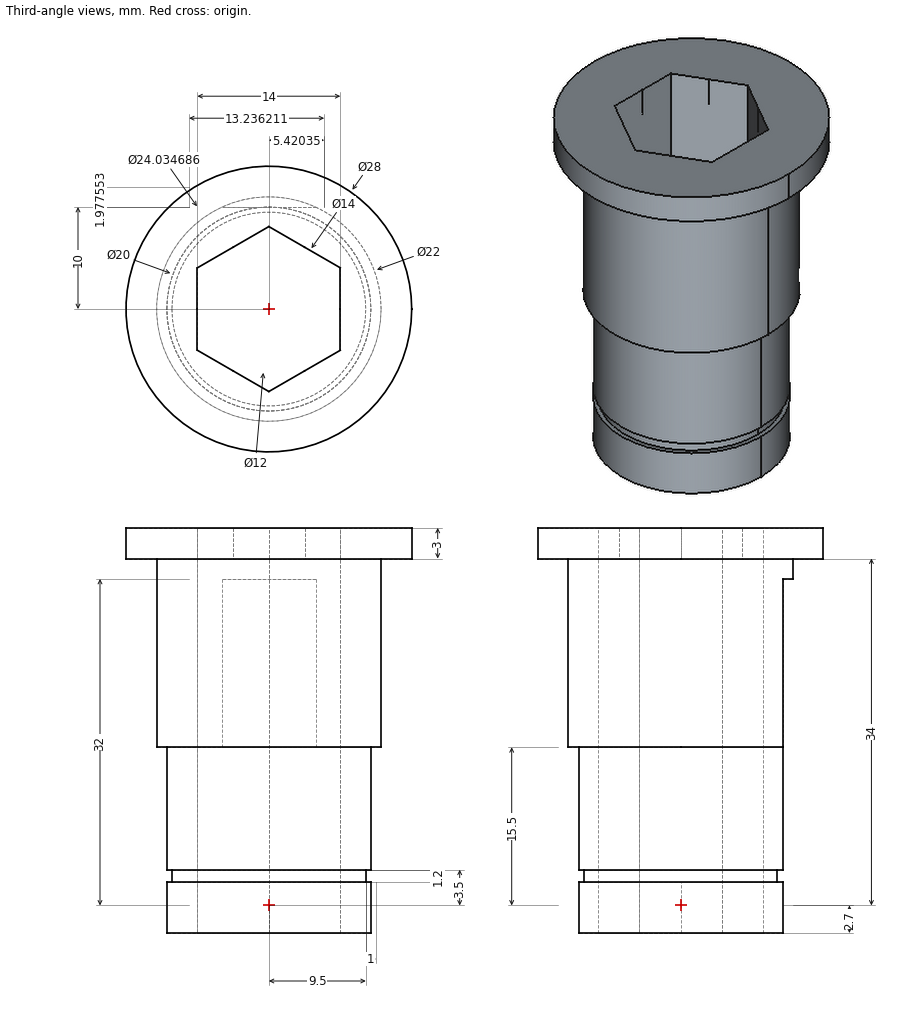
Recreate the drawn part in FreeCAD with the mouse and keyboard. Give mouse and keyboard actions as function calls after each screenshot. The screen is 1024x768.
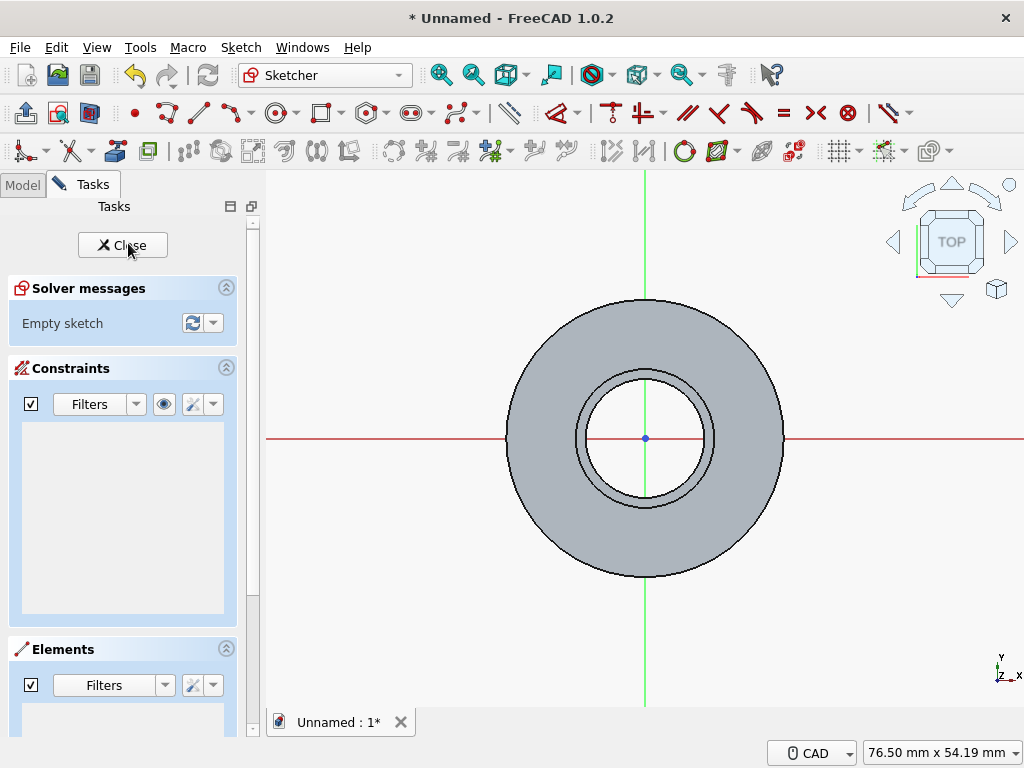
click(90, 114)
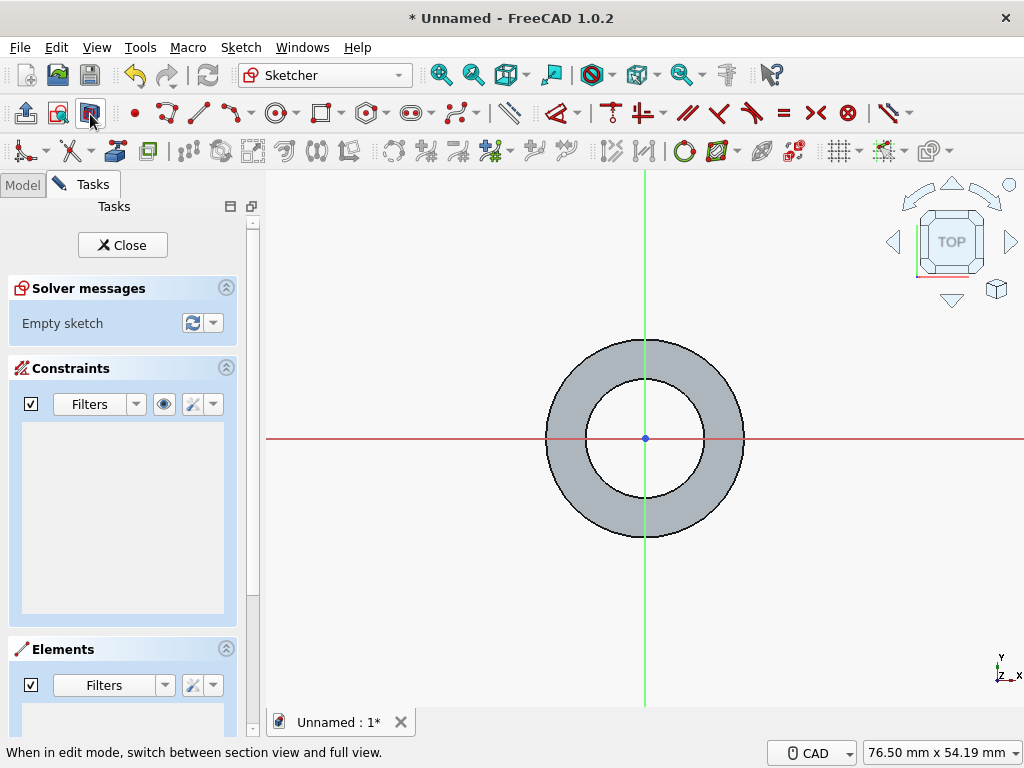
scroll(666, 345, up, 5)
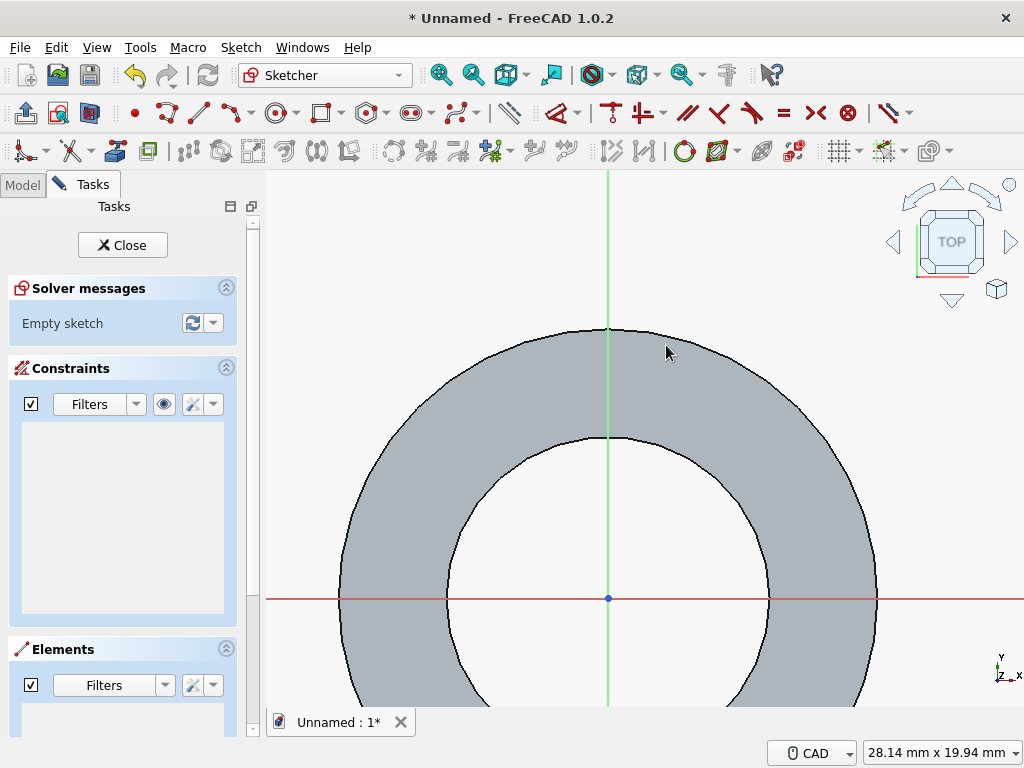
click(322, 114)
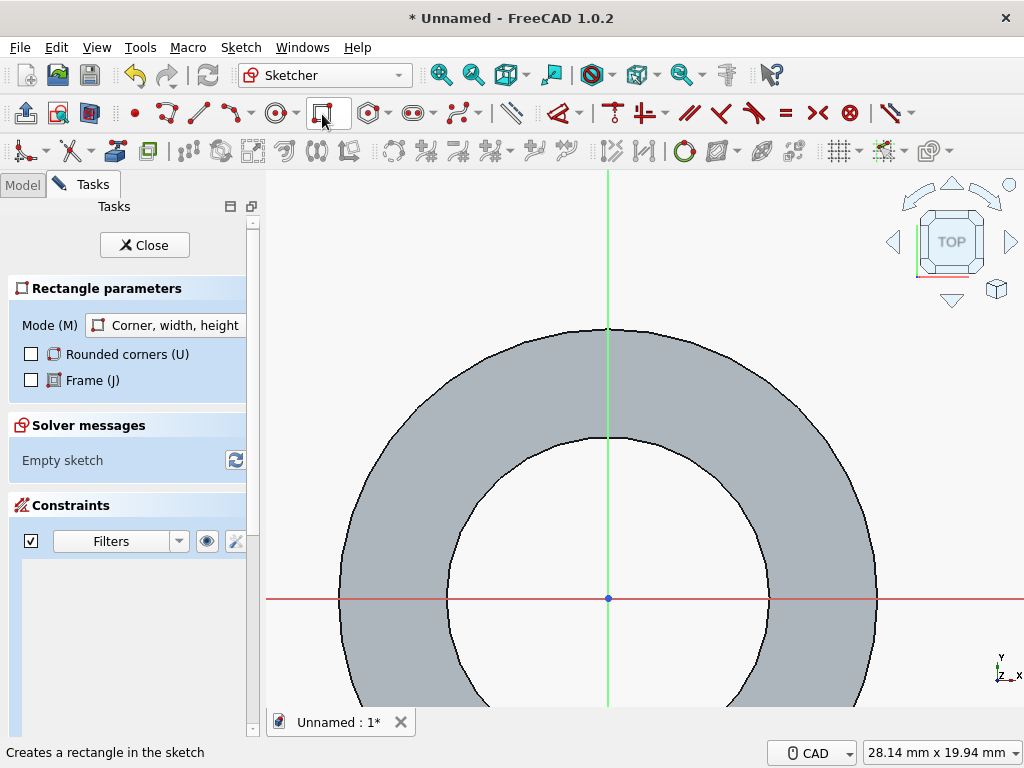
click(397, 276)
click(754, 329)
key(Escape)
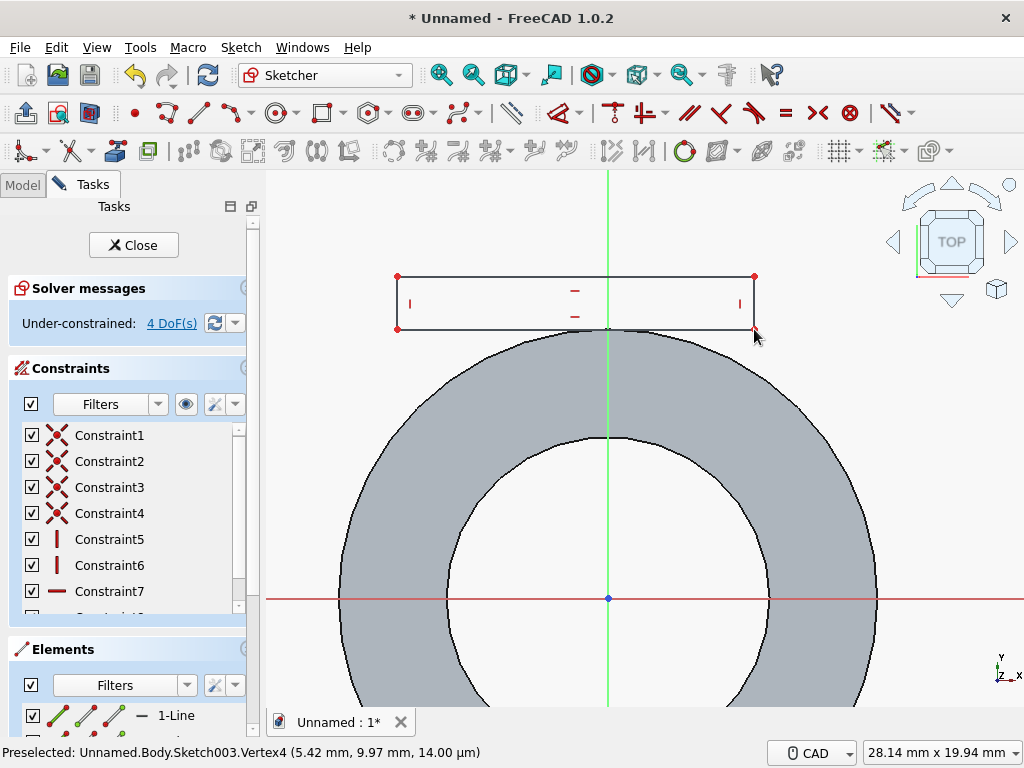
click(558, 114)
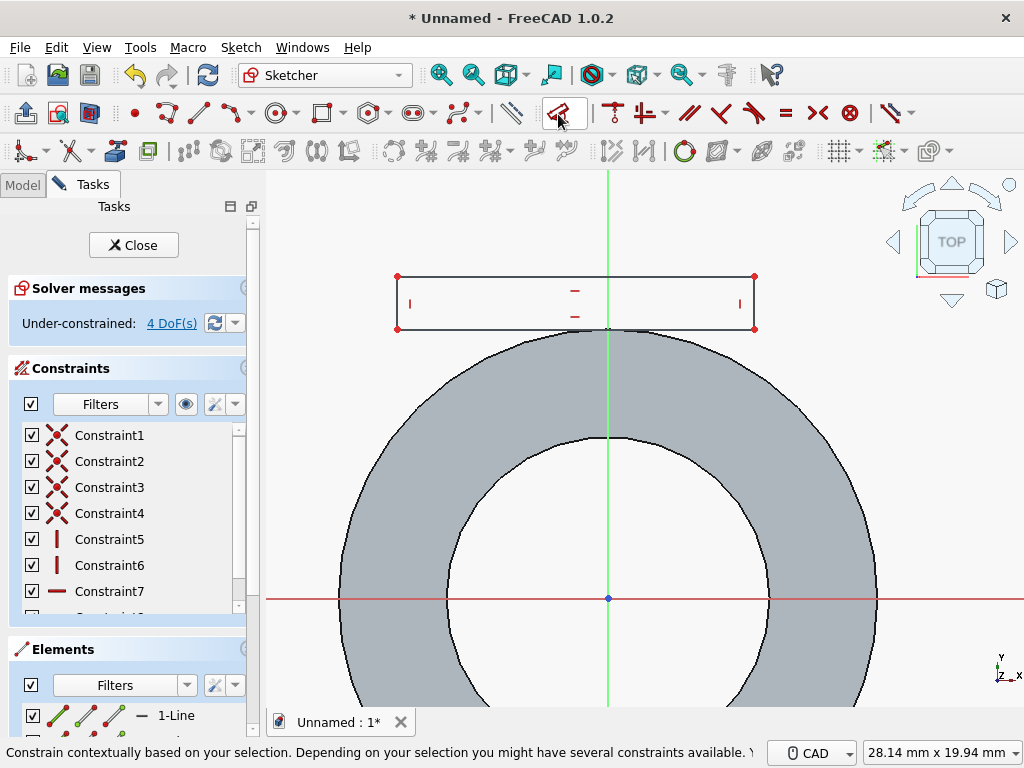
click(397, 330)
click(363, 464)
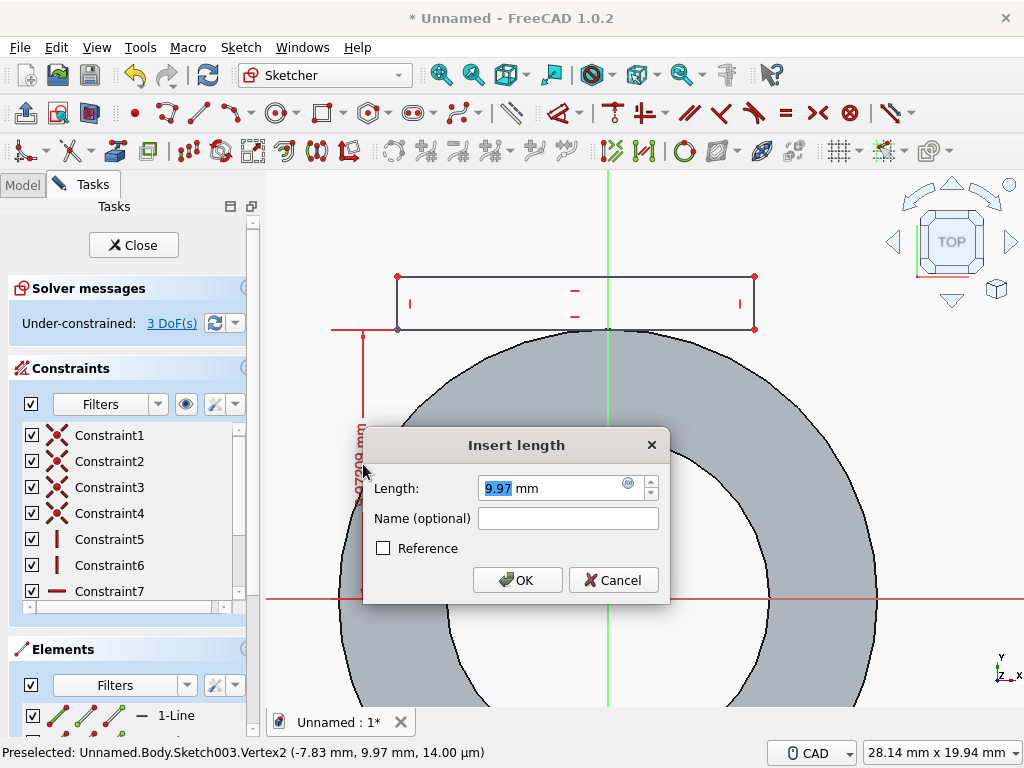
text(10)
key(Return)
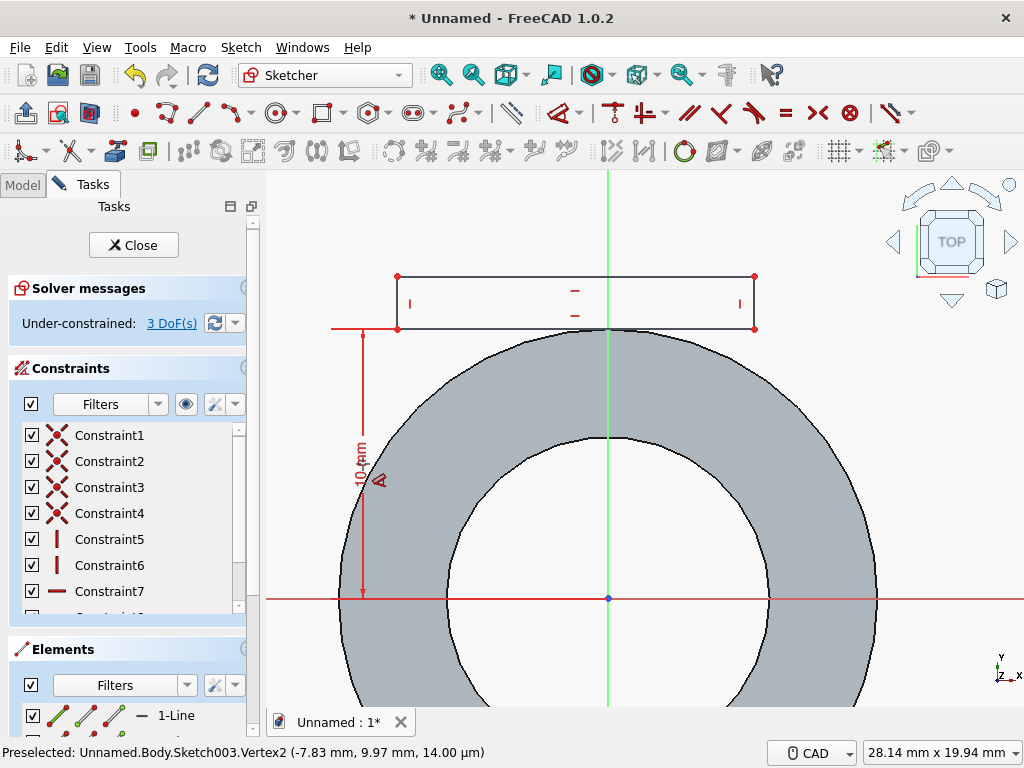
click(397, 293)
click(363, 303)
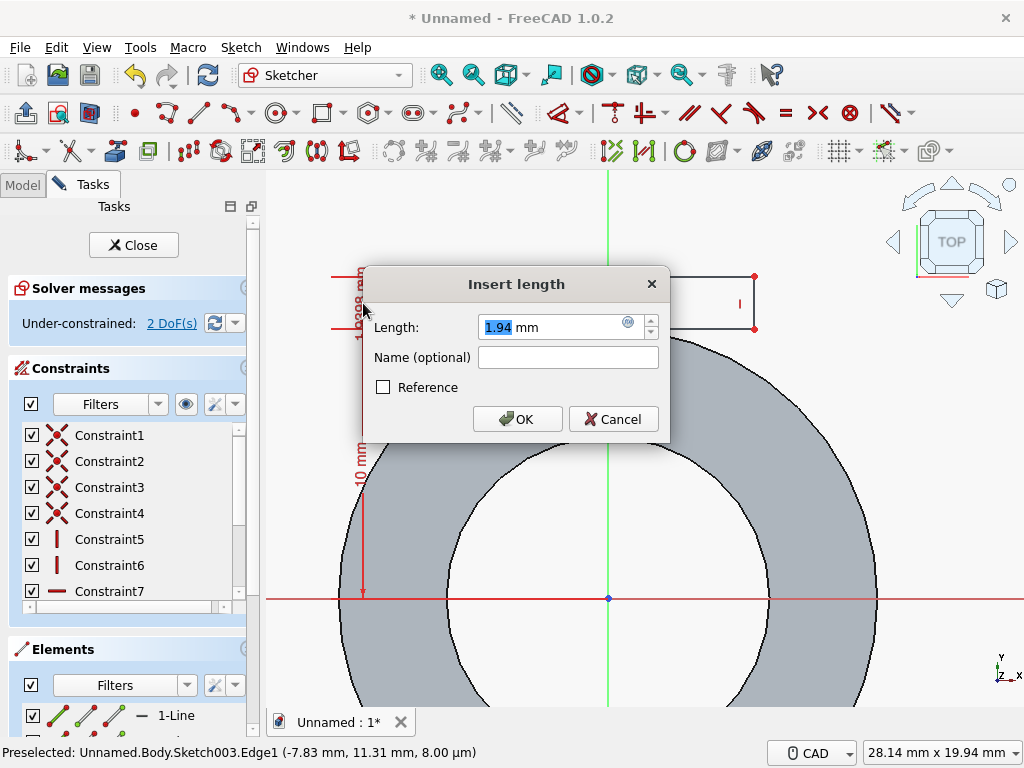
text(1.977553)
key(Return)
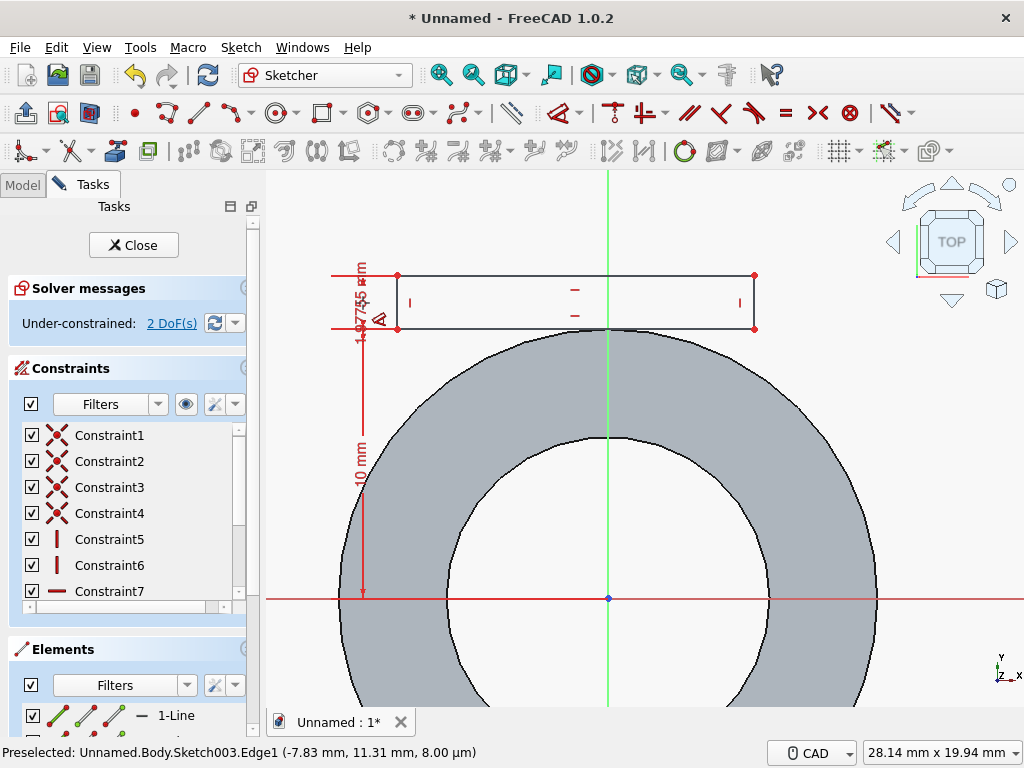
click(754, 329)
click(681, 633)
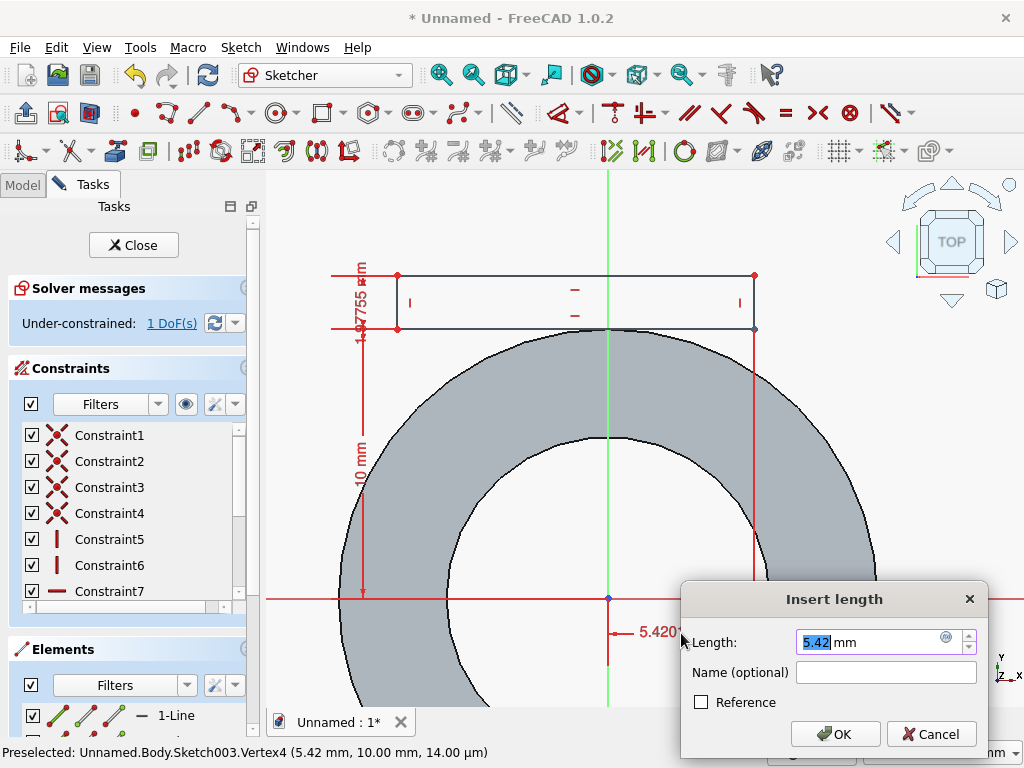
text(5.42035)
key(Return)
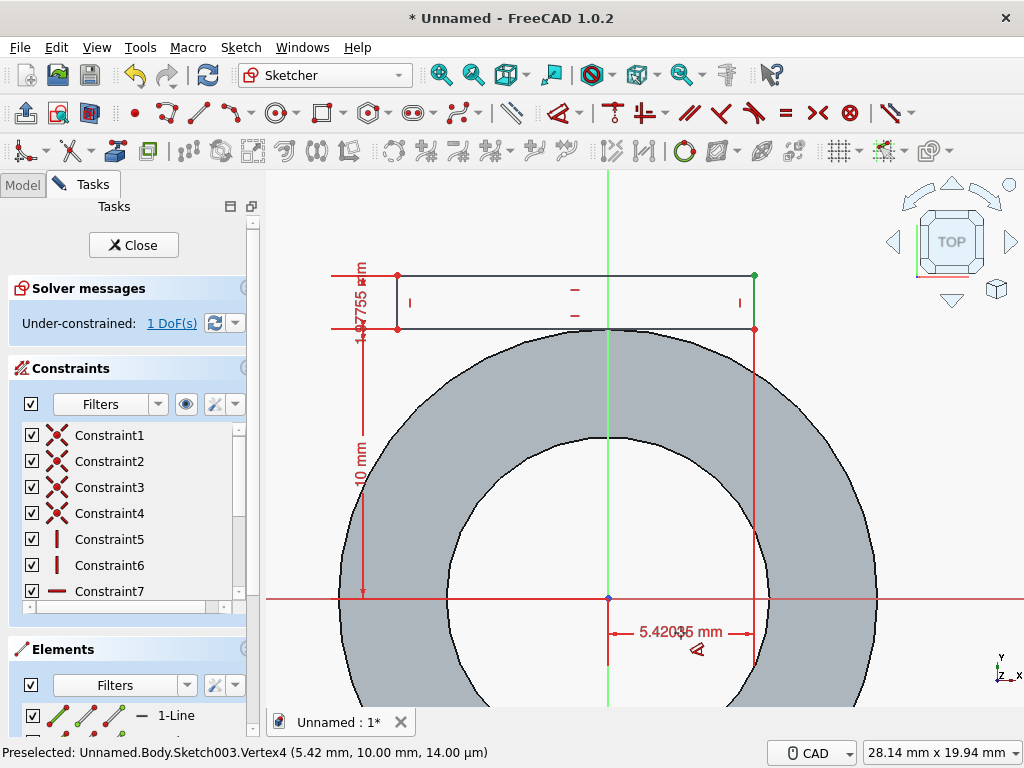
click(504, 329)
click(576, 295)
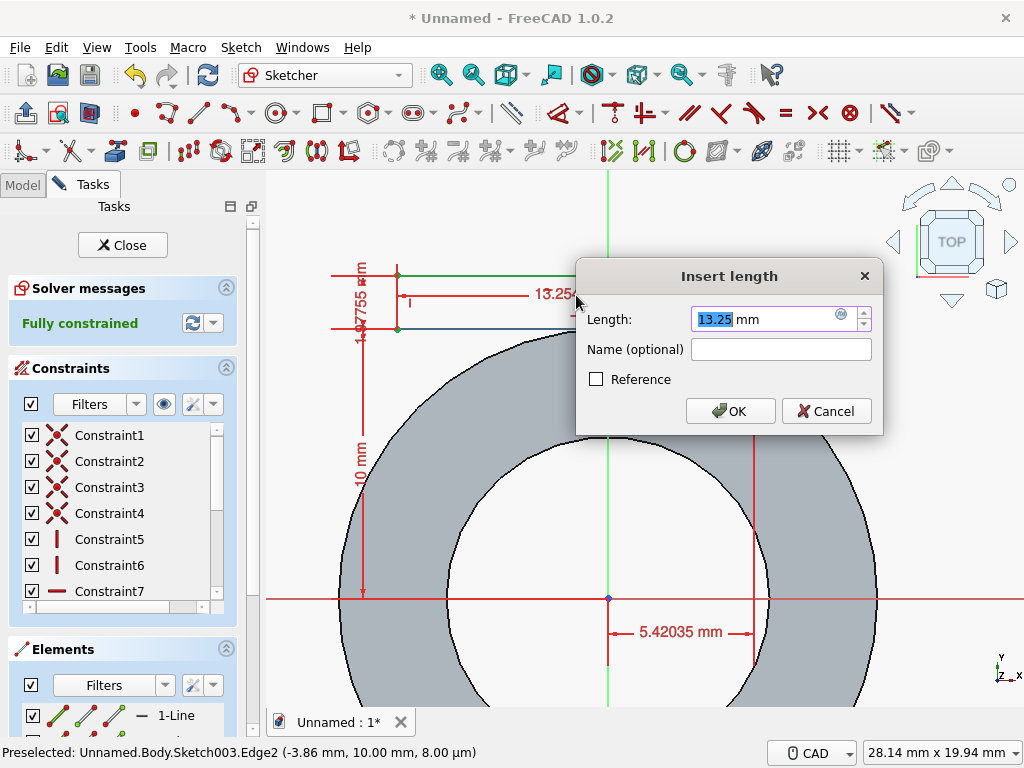
text(13.236211)
key(Return)
key(Escape)